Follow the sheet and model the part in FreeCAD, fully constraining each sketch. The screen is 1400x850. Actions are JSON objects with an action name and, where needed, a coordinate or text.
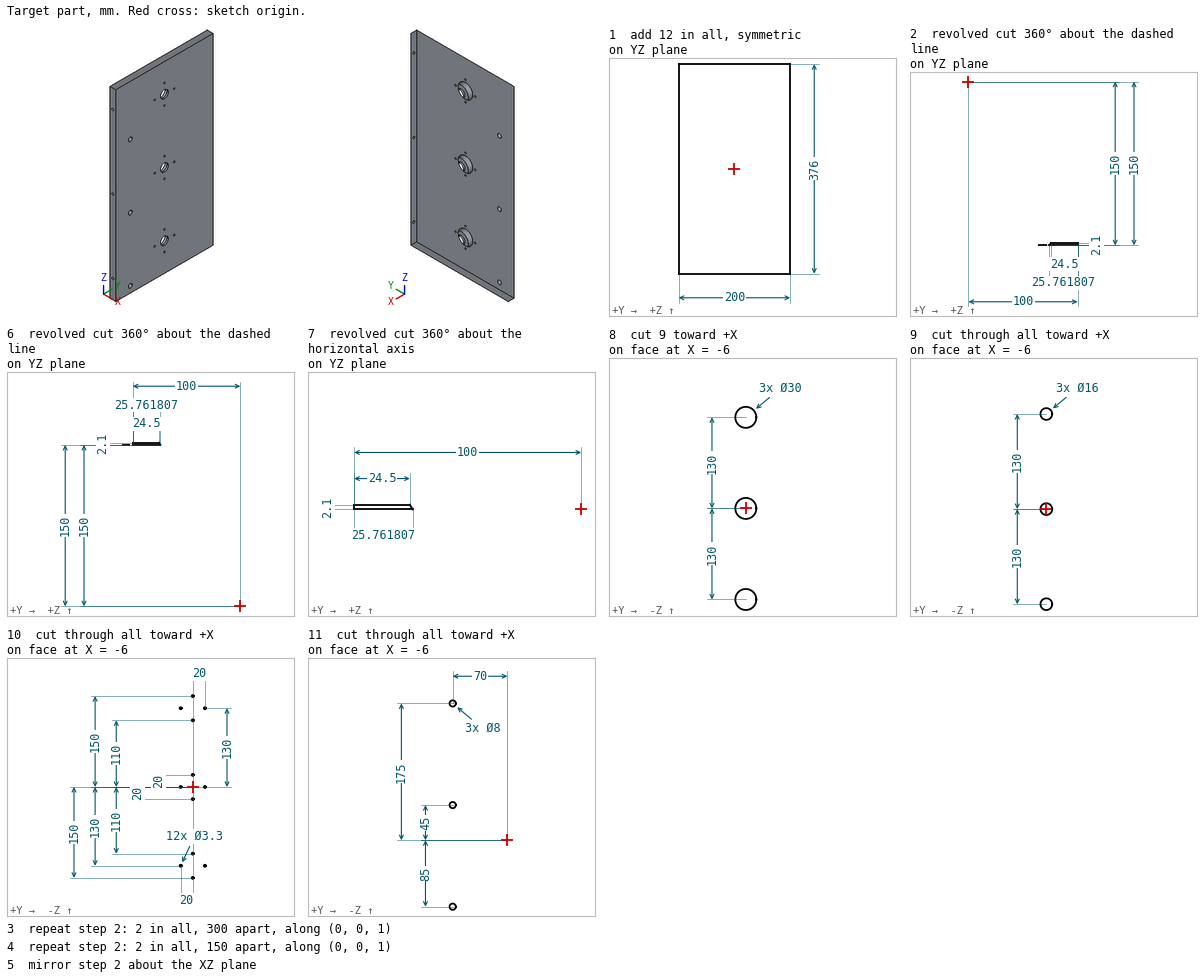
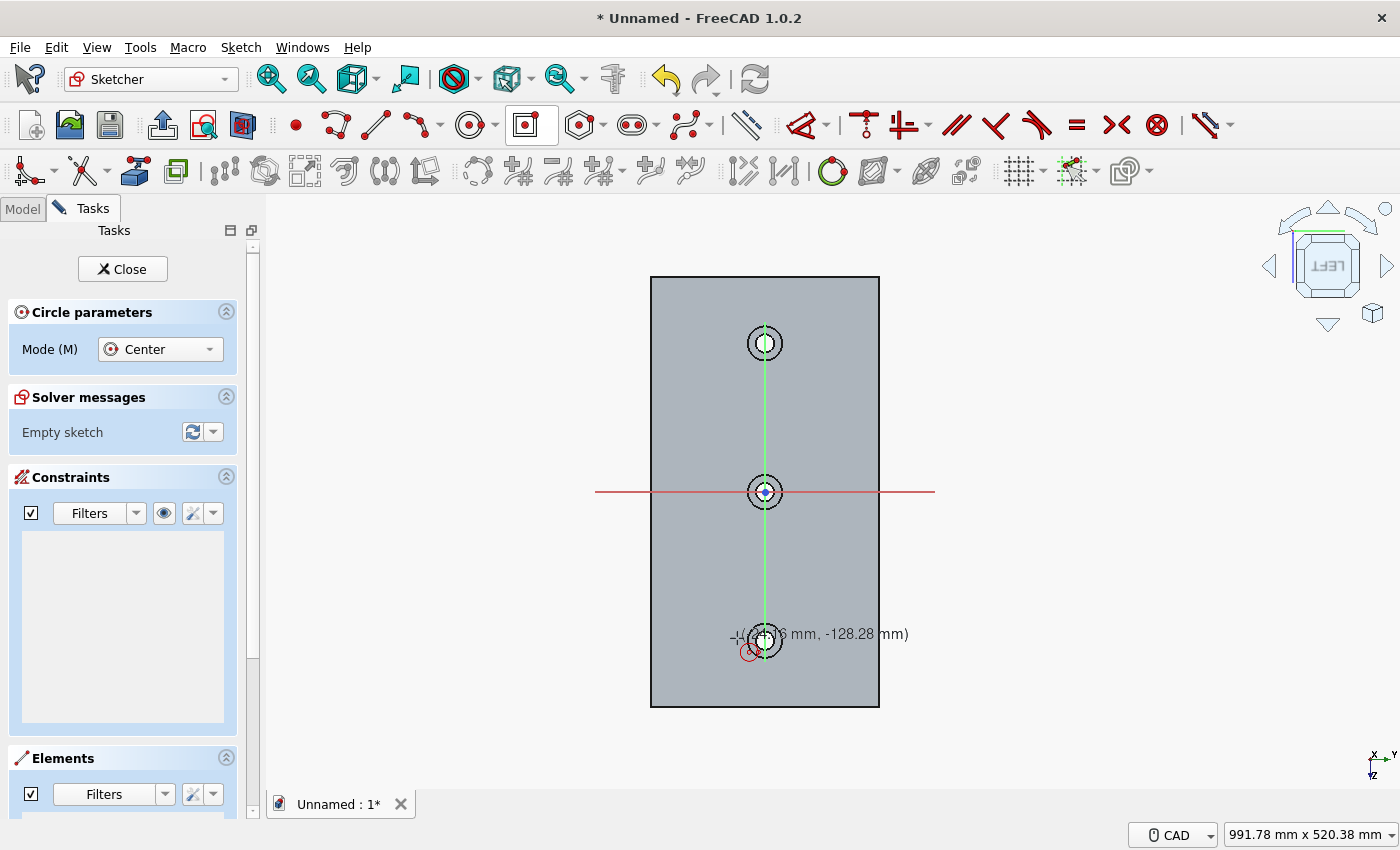
{"action": "left_click", "coordinate": [742, 641]}
{"action": "mouse_move", "coordinate": [743, 639]}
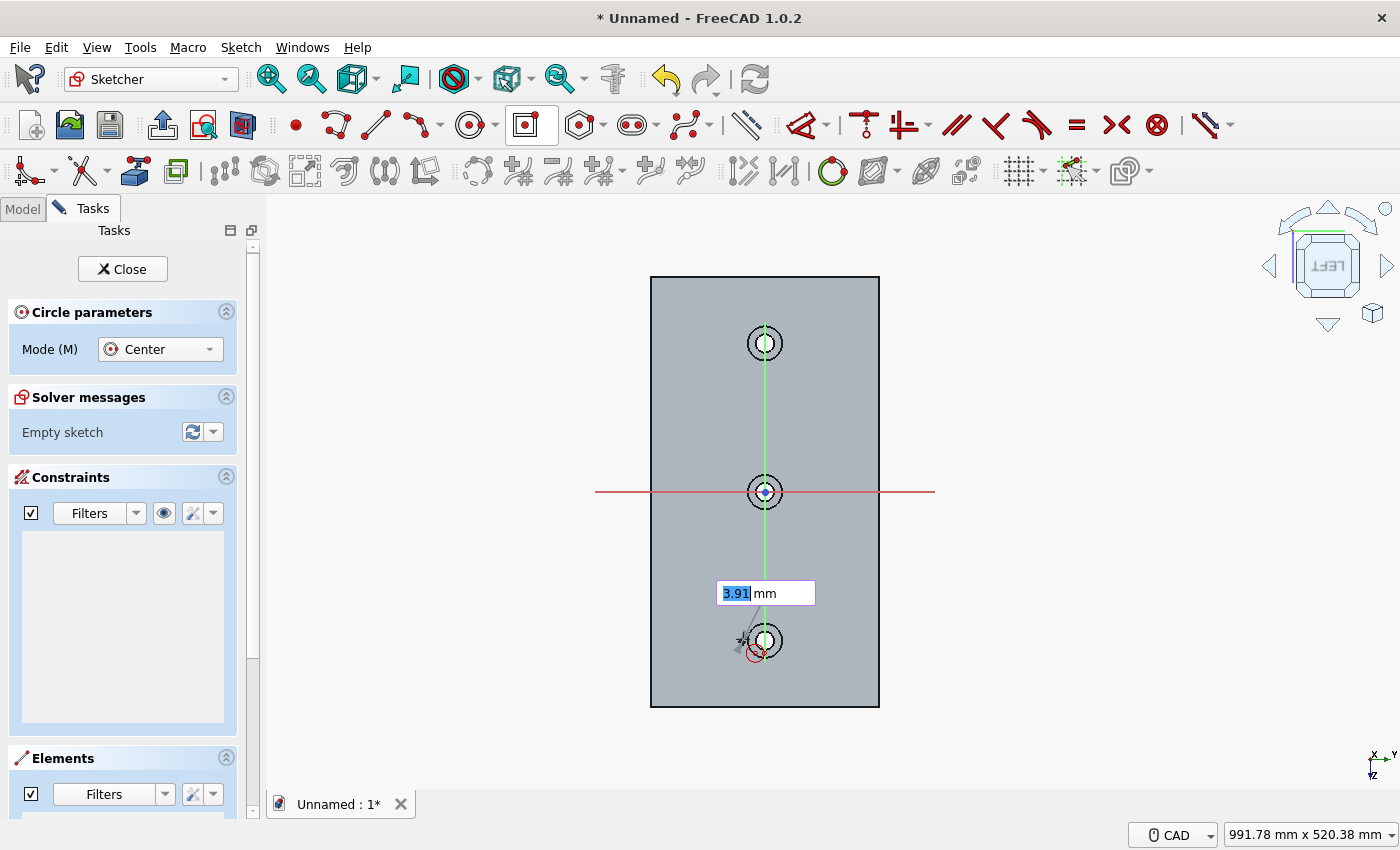
{"action": "type", "text": "3.3"}
{"action": "key", "text": "Return"}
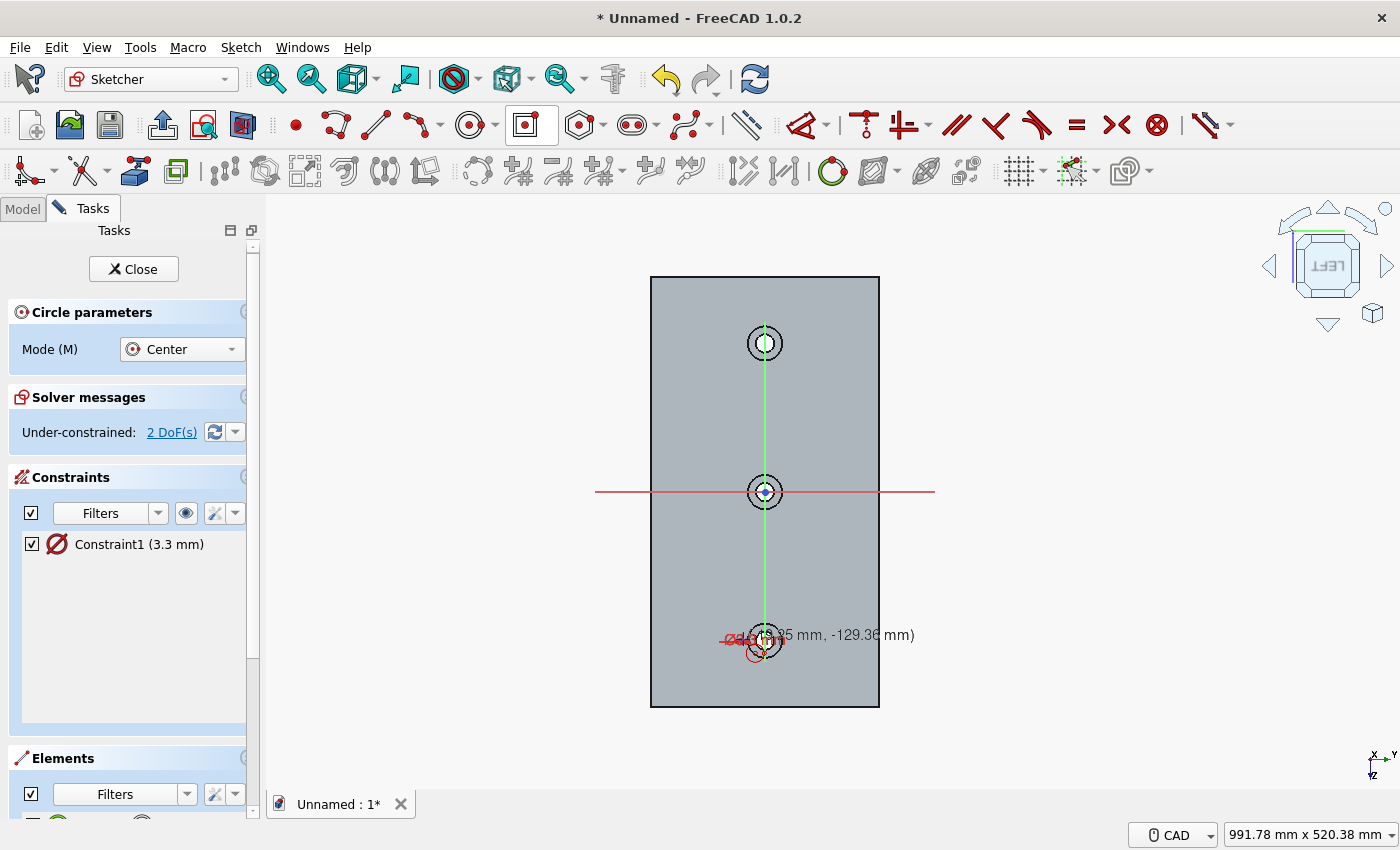
{"action": "scroll", "coordinate": [765, 321], "scroll_direction": "up", "scroll_amount": 13}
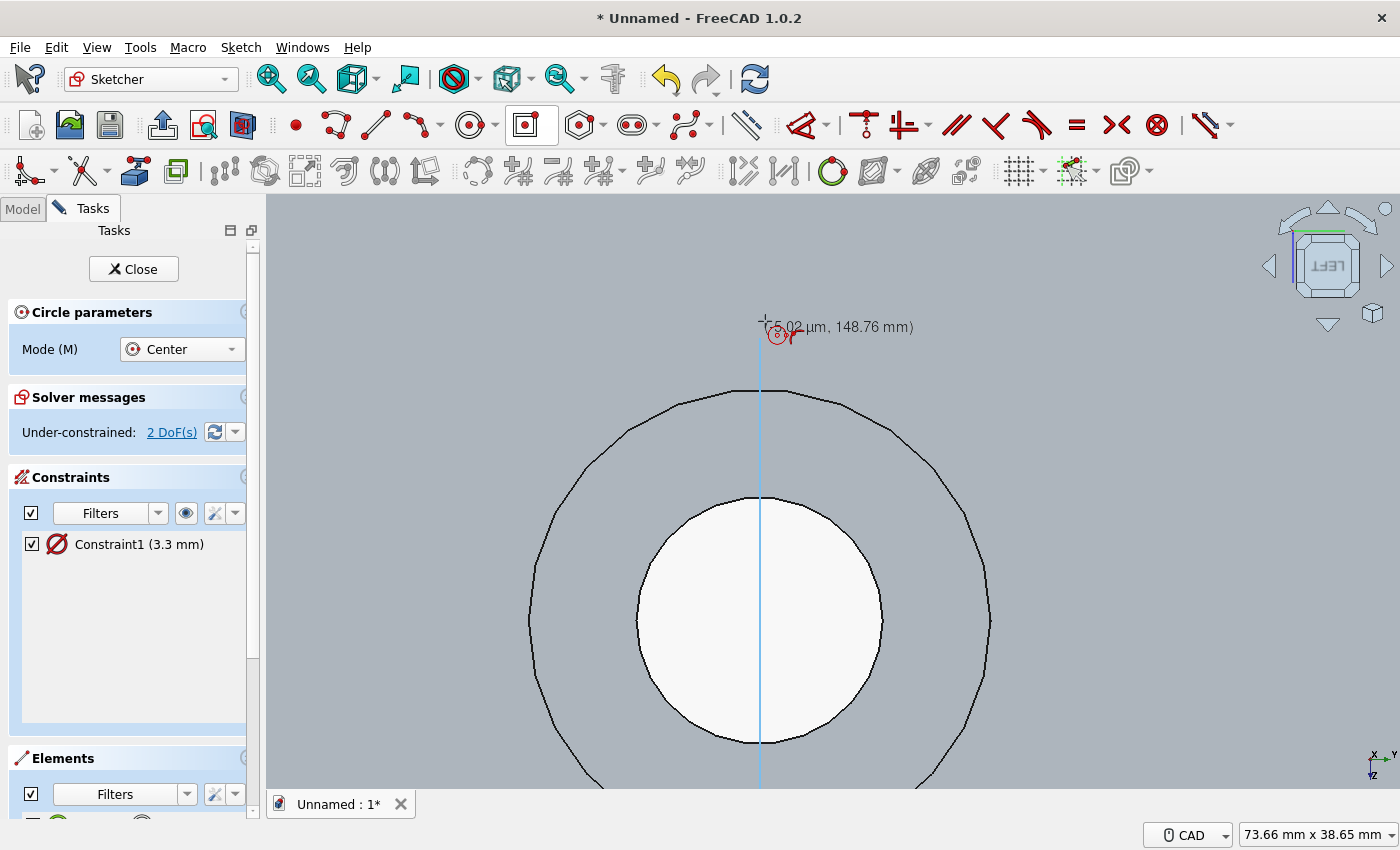
{"action": "scroll", "coordinate": [765, 321], "scroll_direction": "down", "scroll_amount": 13}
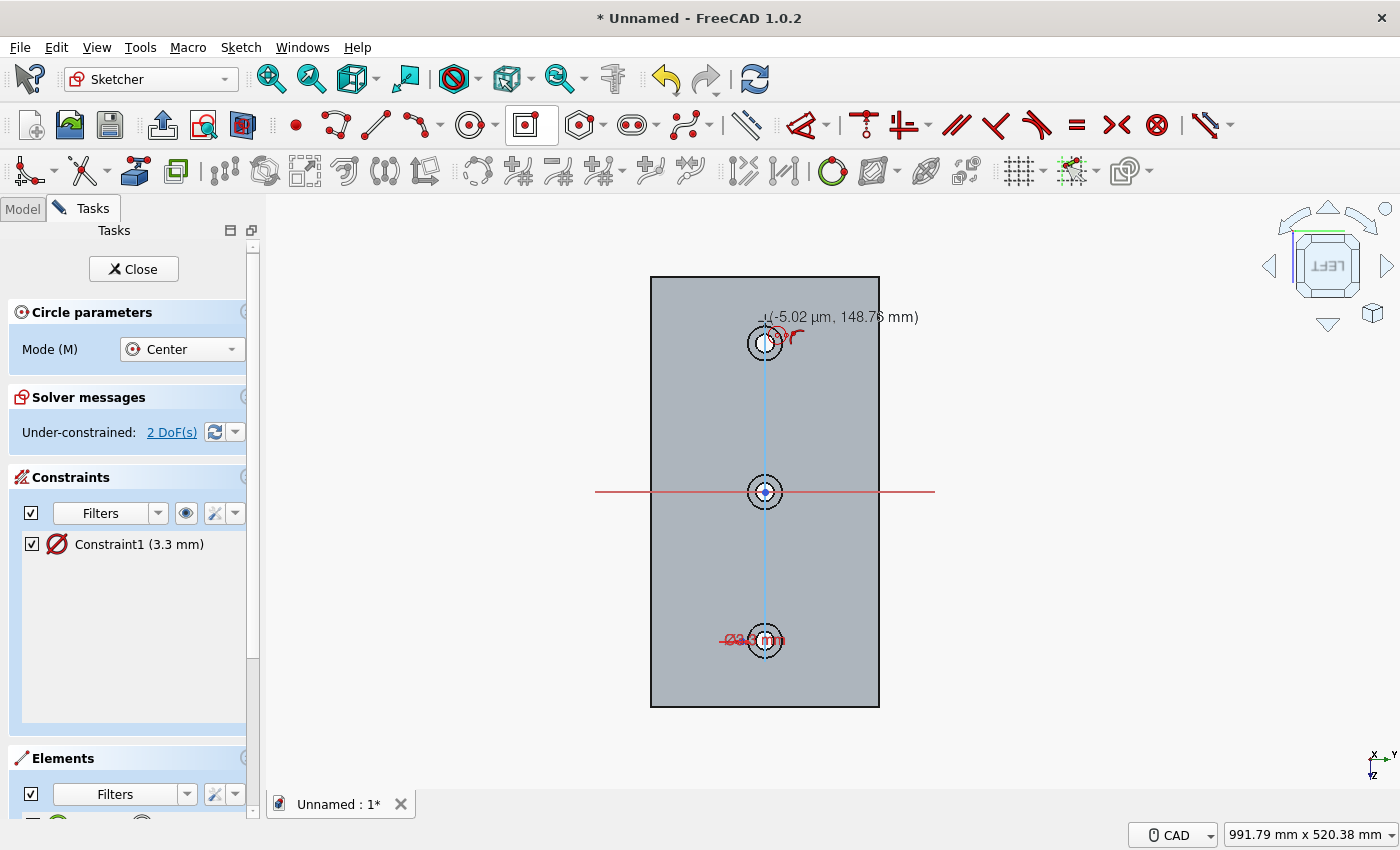
{"action": "left_click", "coordinate": [765, 321]}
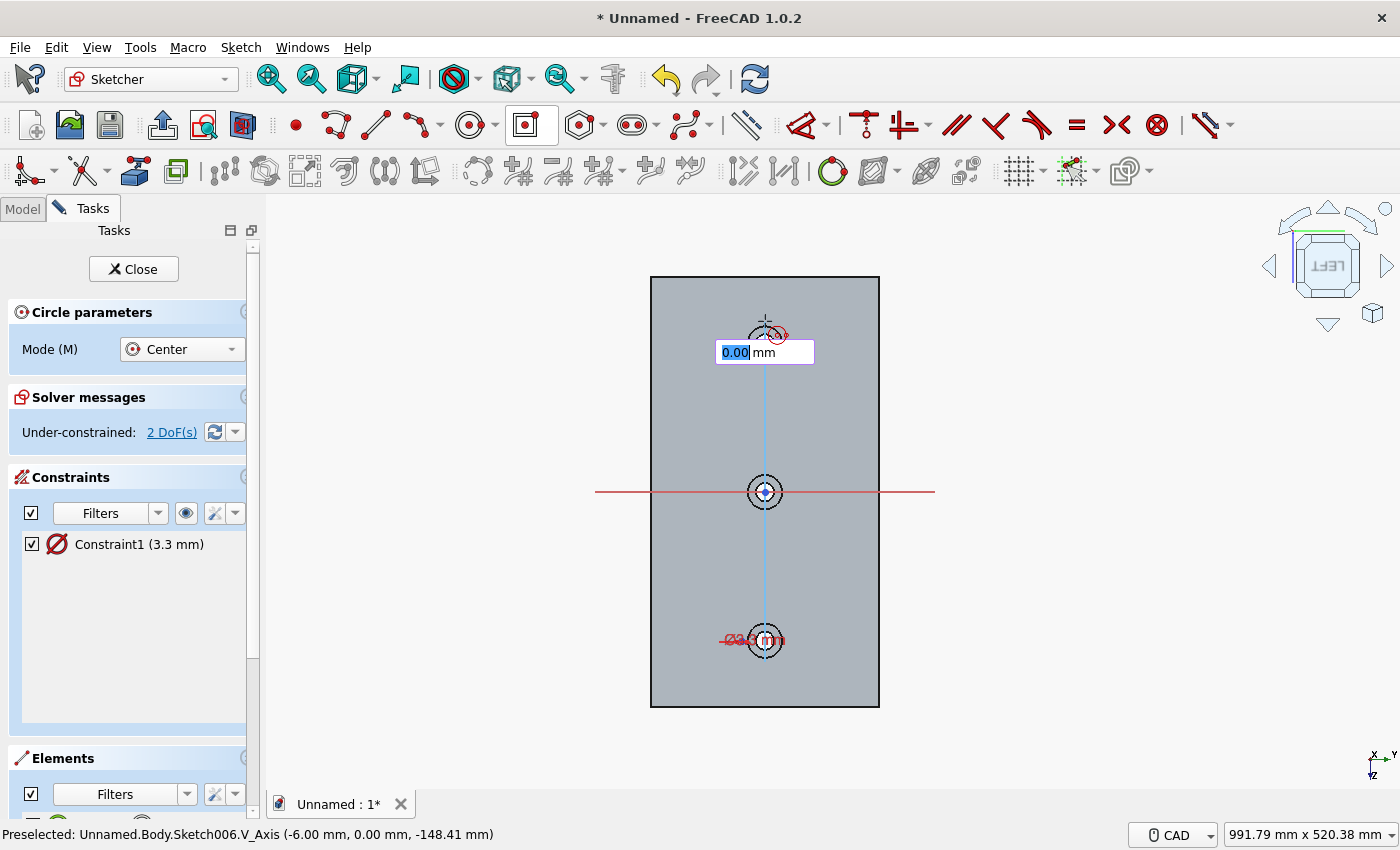
{"action": "scroll", "coordinate": [767, 320], "scroll_direction": "up", "scroll_amount": 11}
{"action": "mouse_move", "coordinate": [761, 318]}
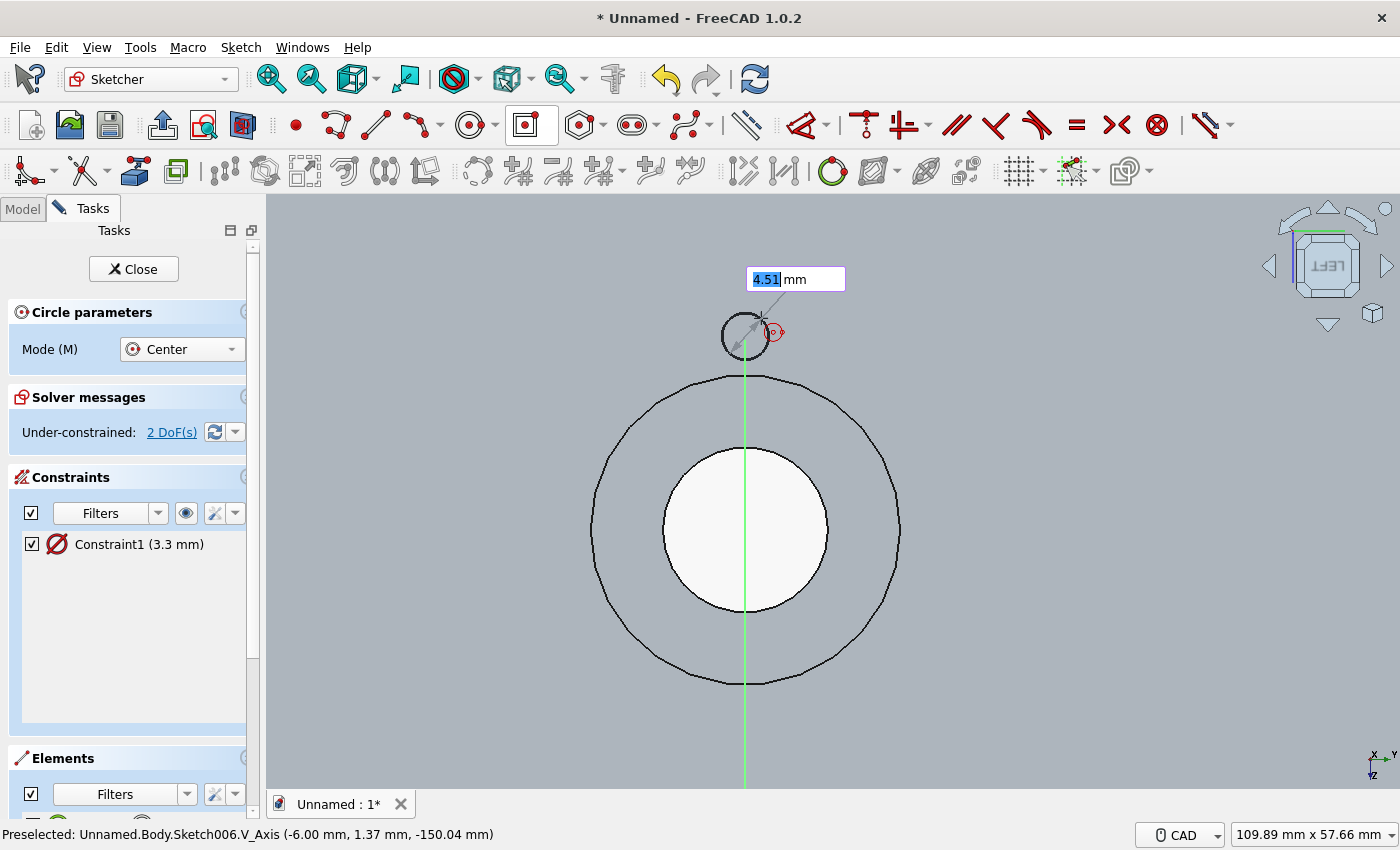
{"action": "type", "text": "3.3"}
{"action": "key", "text": "Return"}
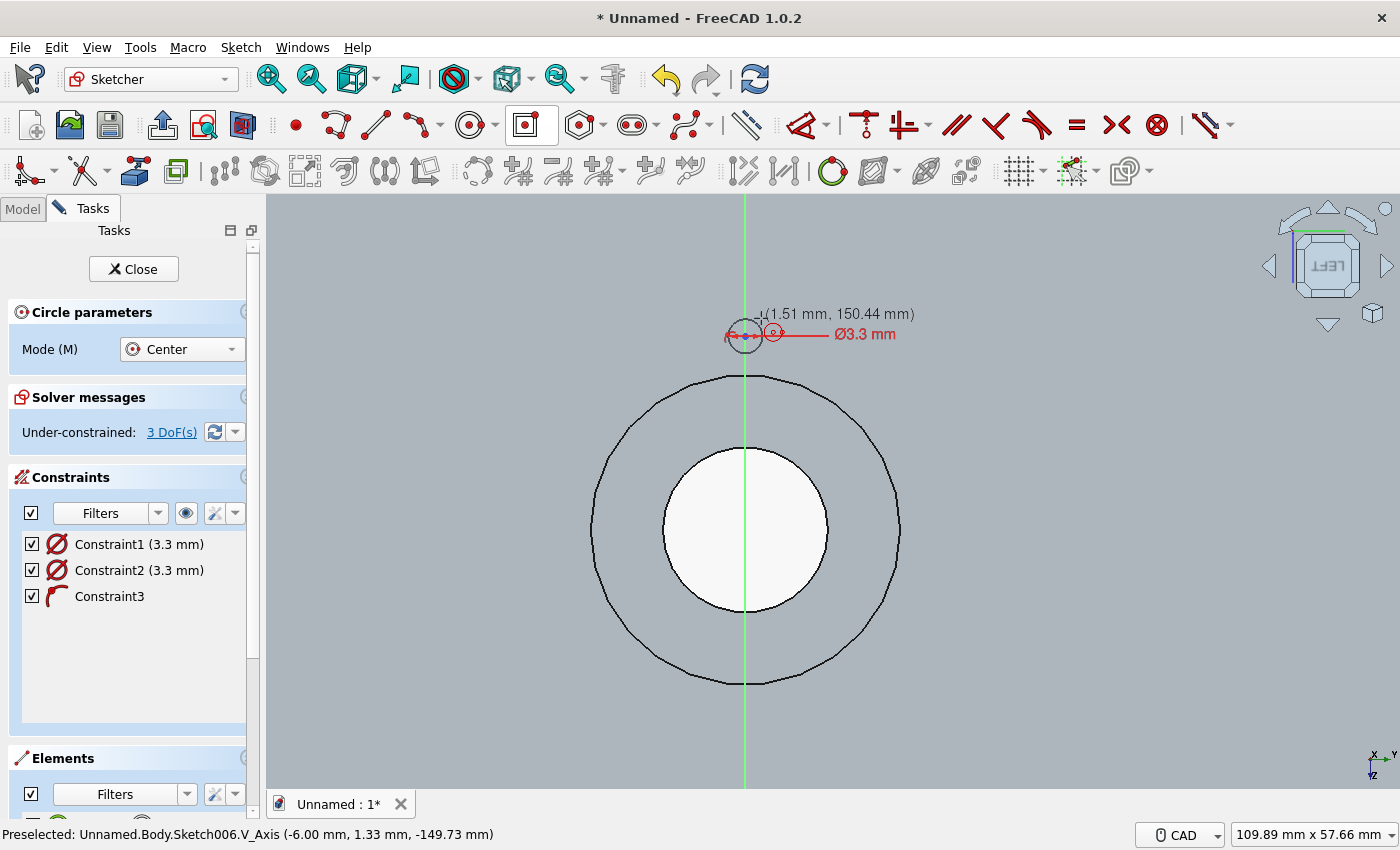
{"action": "scroll", "coordinate": [952, 530], "scroll_direction": "up", "scroll_amount": 2}